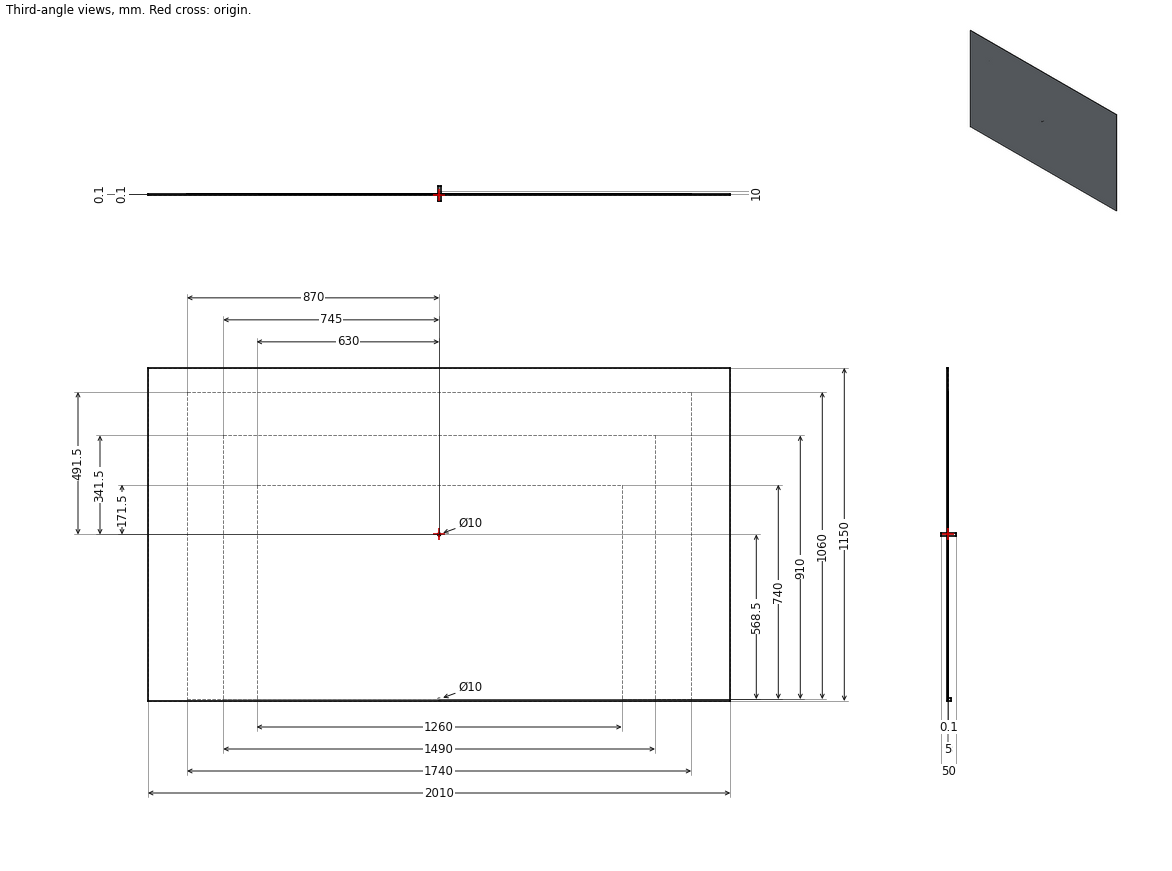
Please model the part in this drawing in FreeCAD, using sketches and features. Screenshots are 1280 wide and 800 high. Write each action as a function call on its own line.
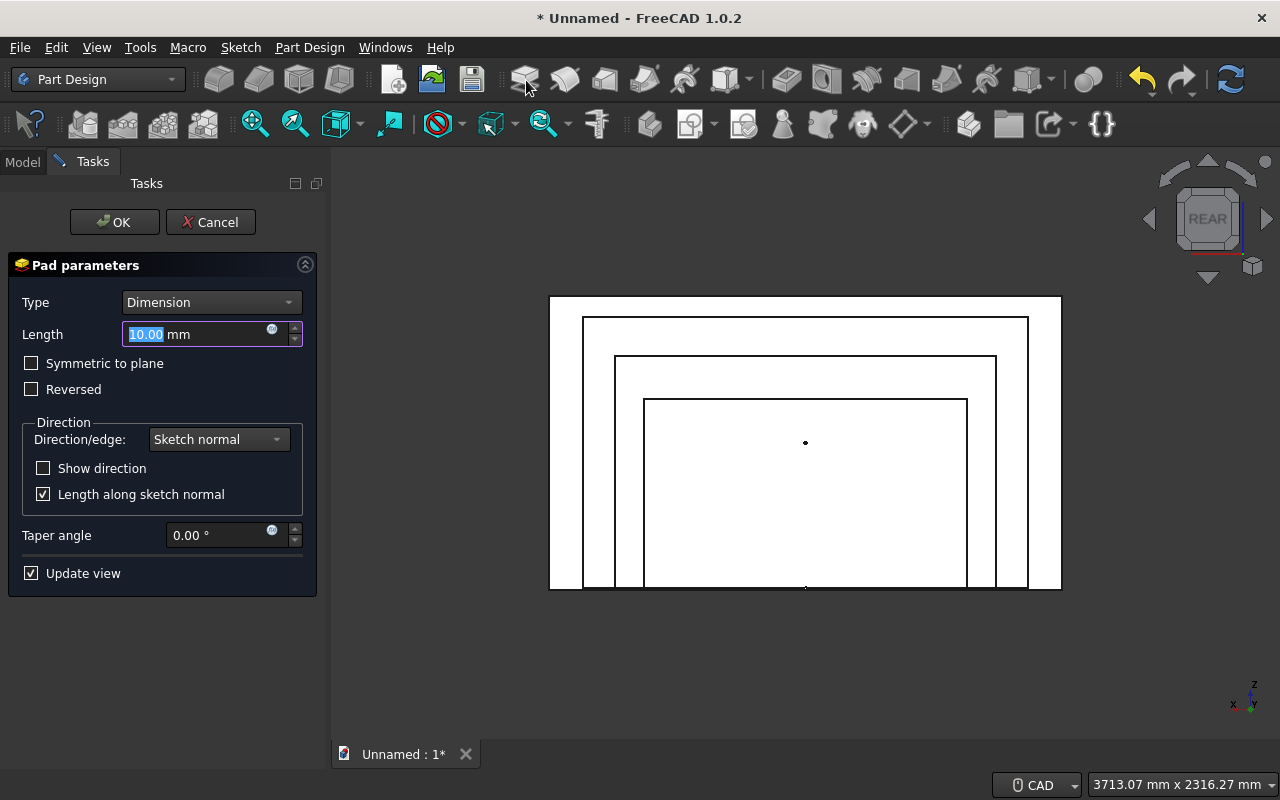
text(10)
key(Tab)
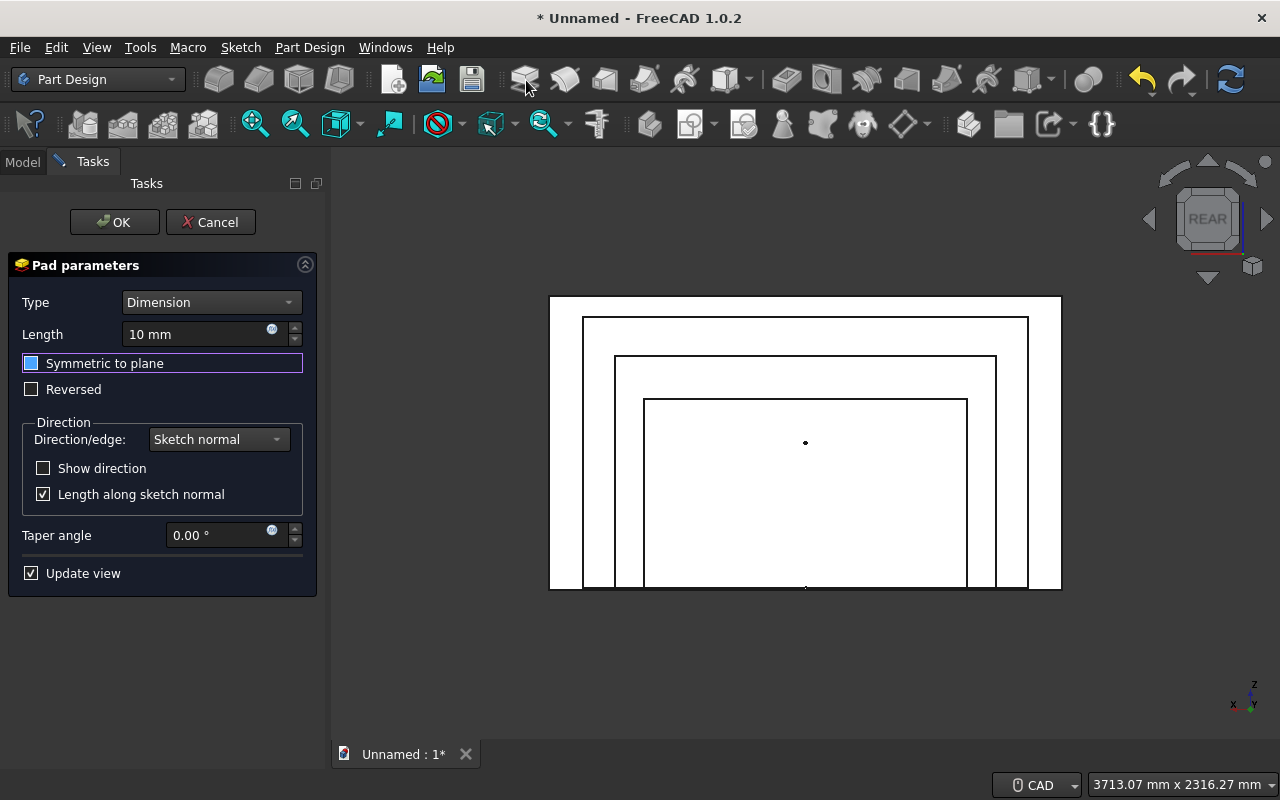
click(115, 222)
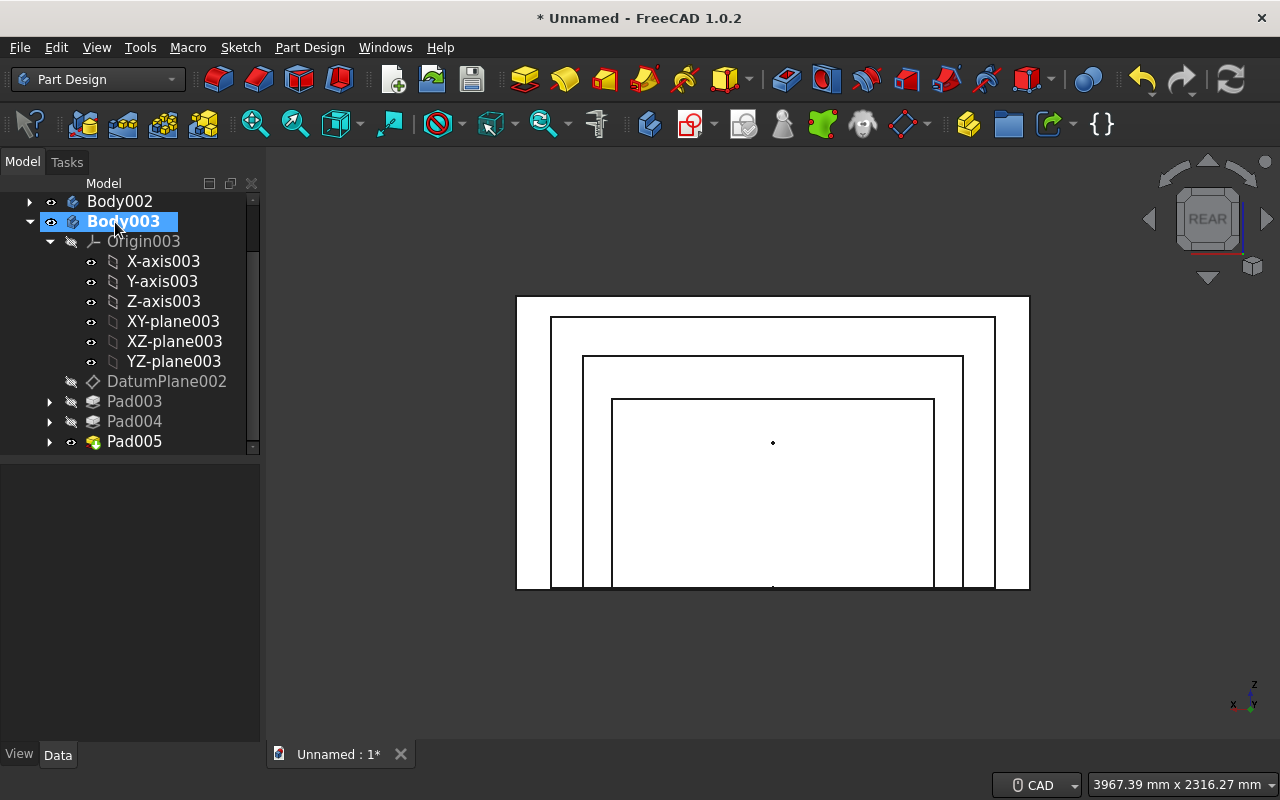
key(0)